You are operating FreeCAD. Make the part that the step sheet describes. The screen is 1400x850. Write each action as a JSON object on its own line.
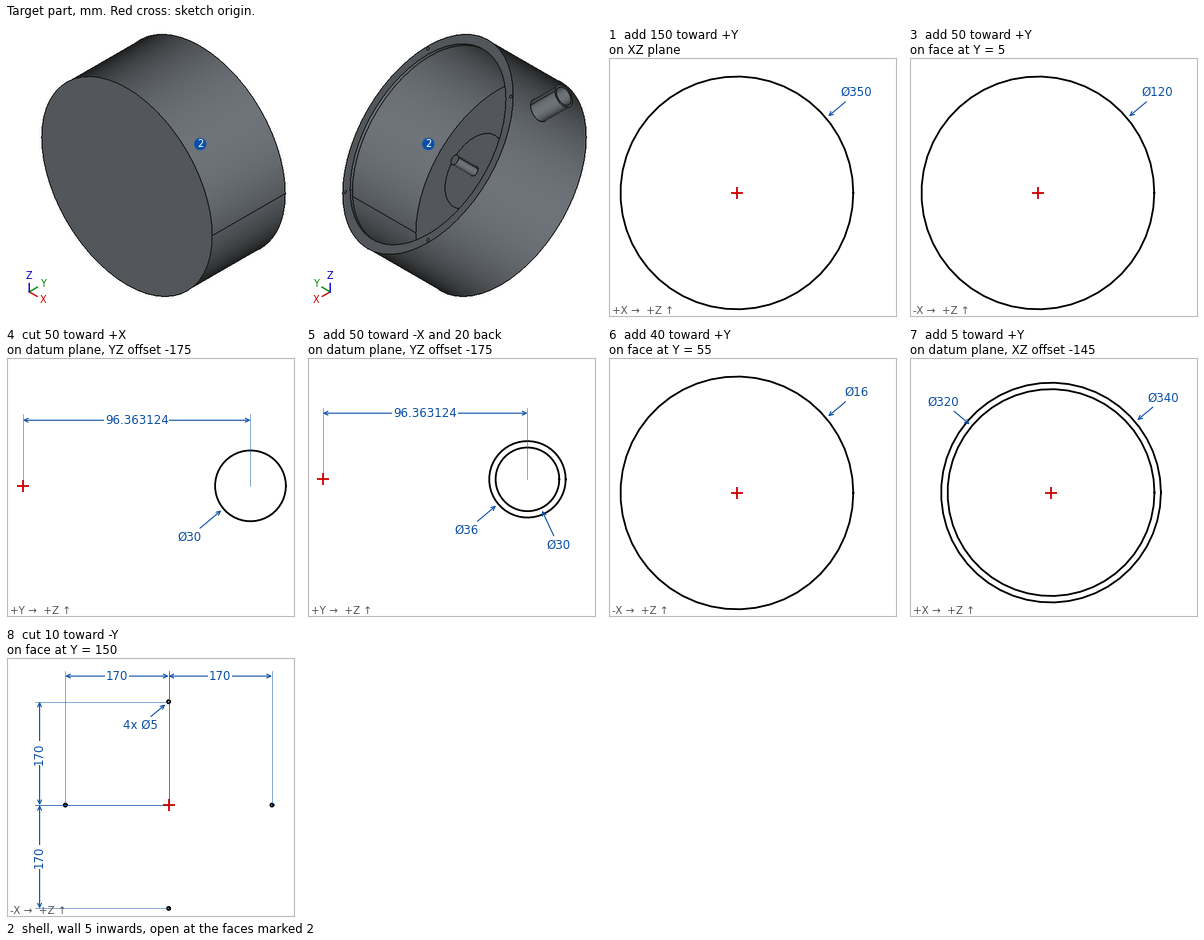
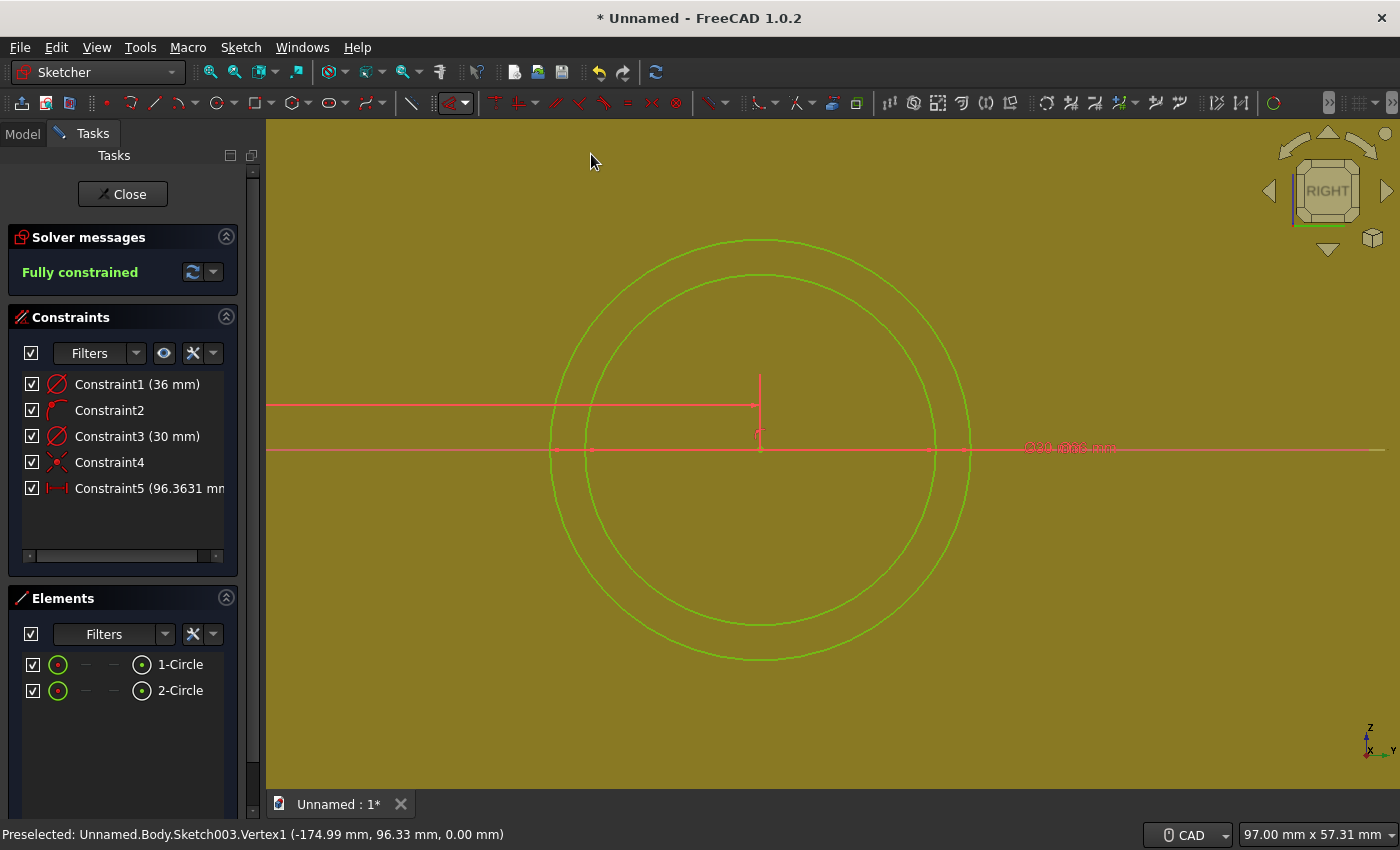
{"action": "left_click", "coordinate": [123, 194]}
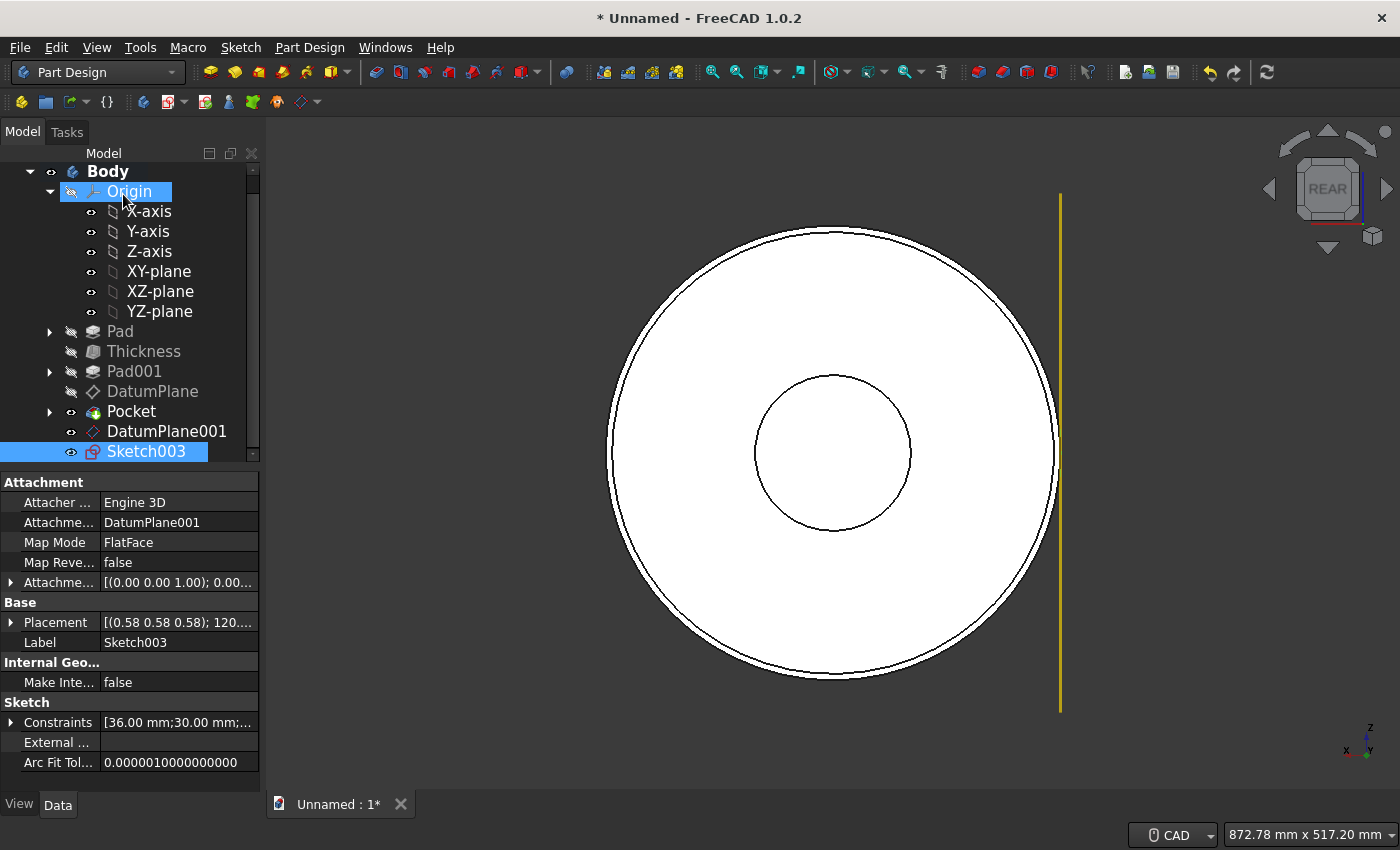
{"action": "left_click", "coordinate": [212, 72]}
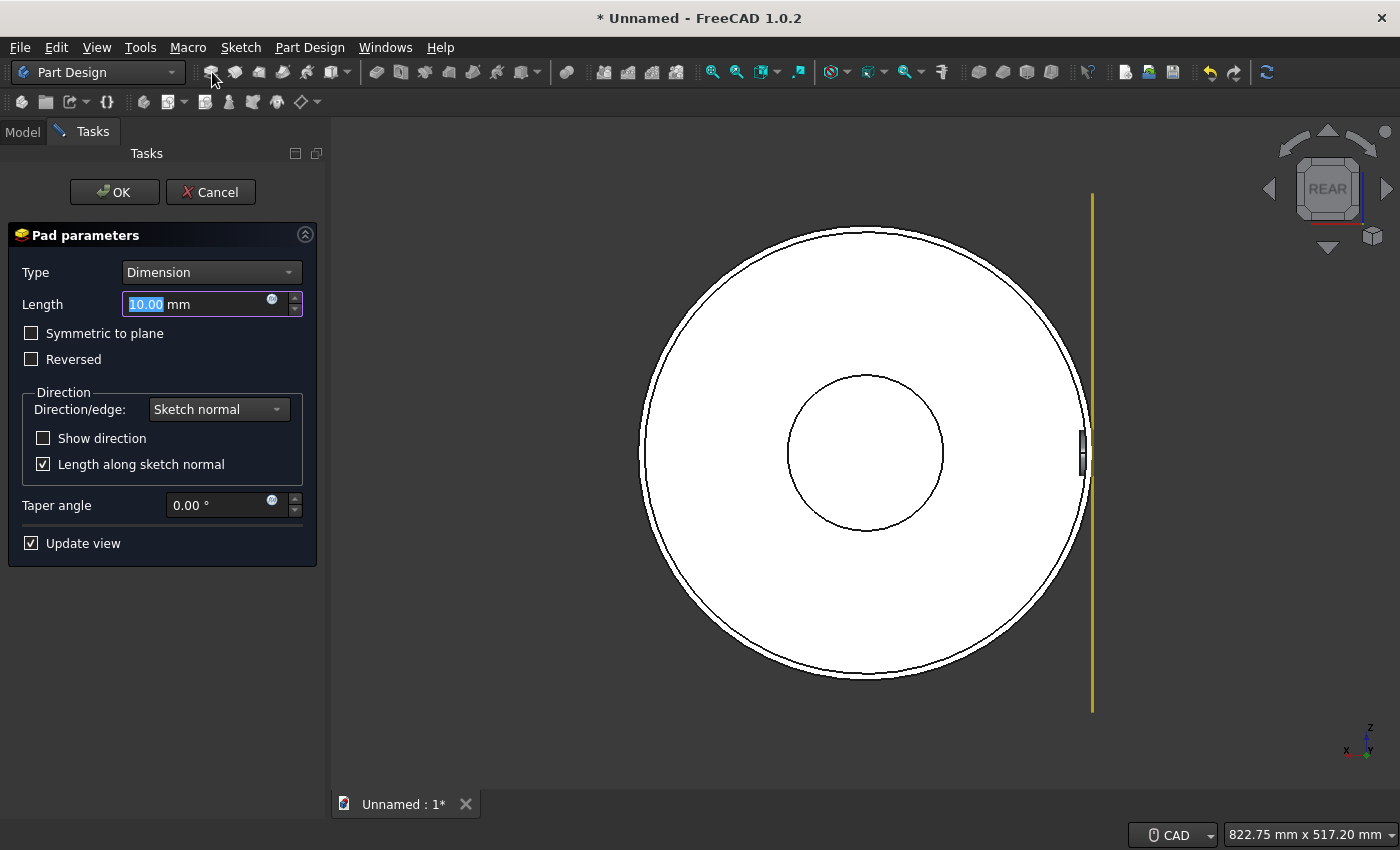
{"action": "left_click", "coordinate": [212, 272]}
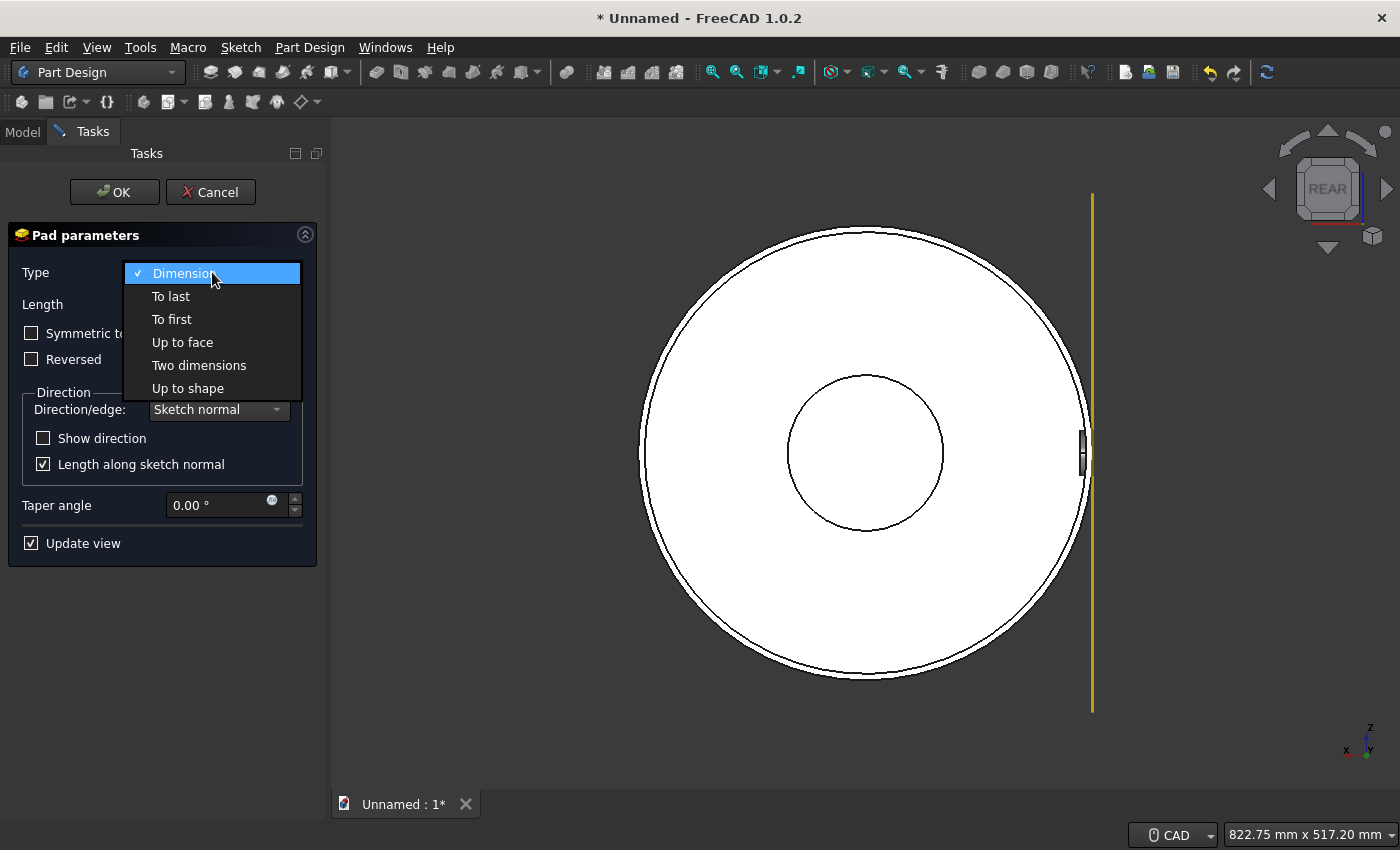
{"action": "left_click", "coordinate": [212, 366]}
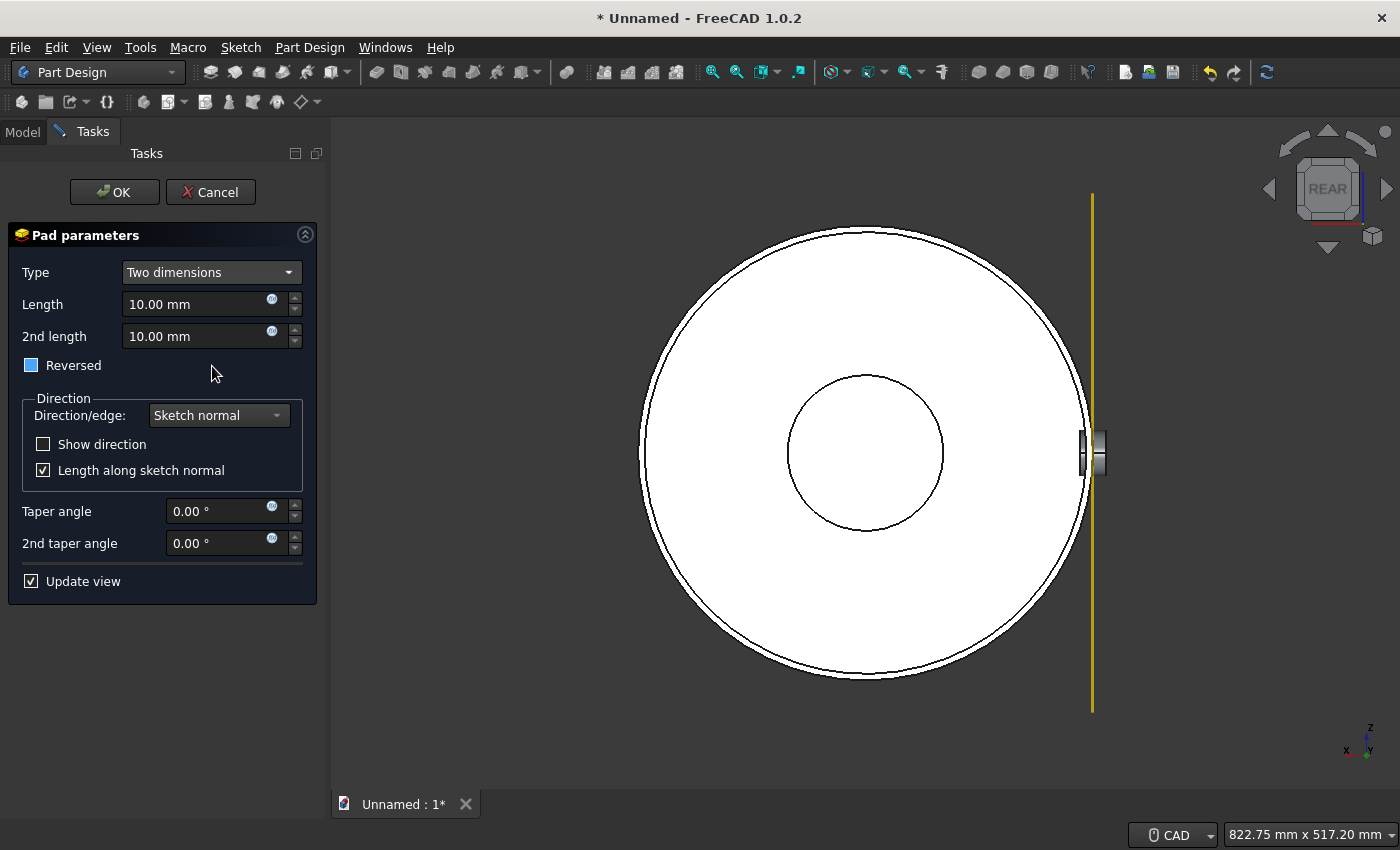
{"action": "triple_click", "coordinate": [204, 304]}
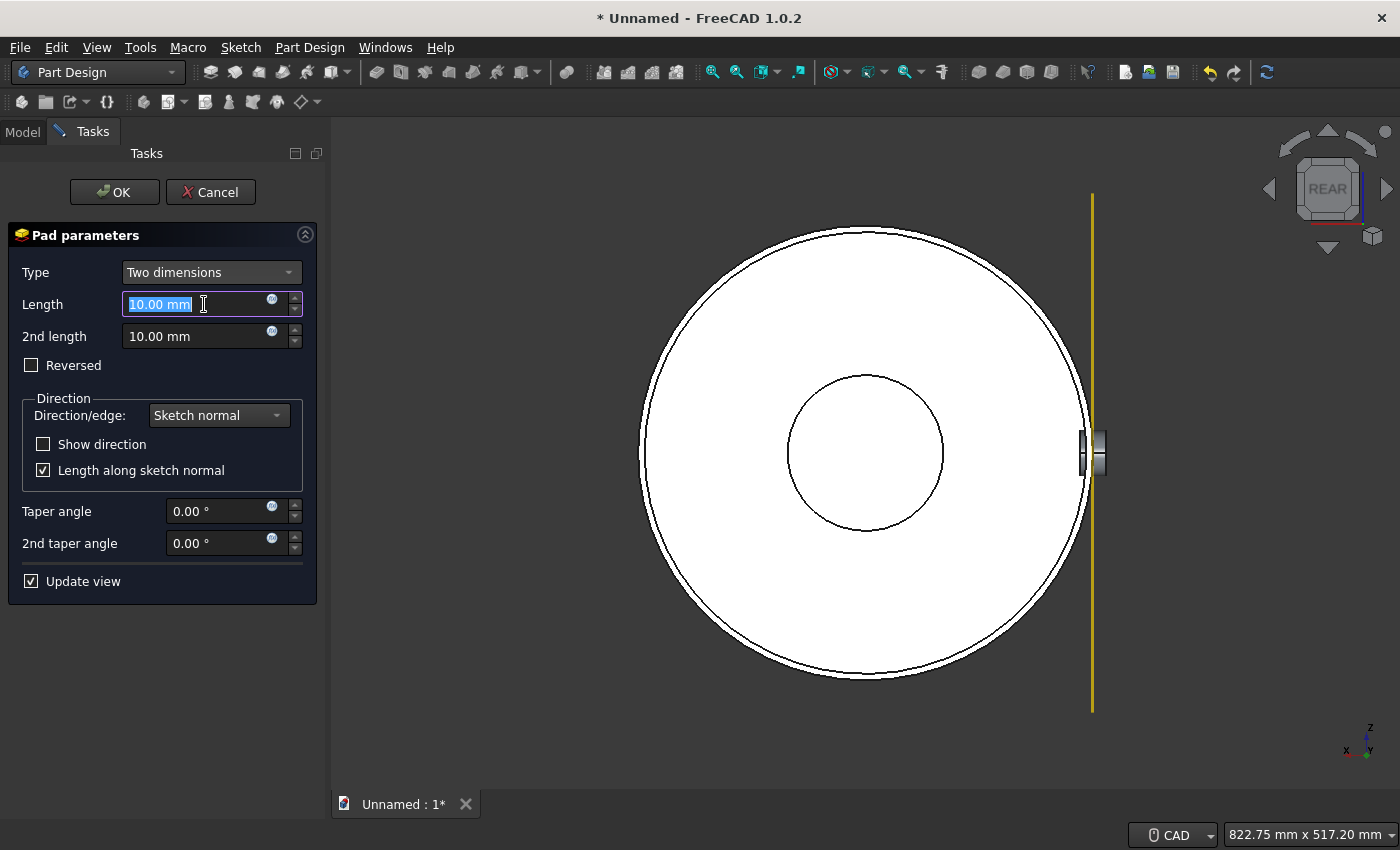
{"action": "type", "text": "50"}
{"action": "key", "text": "Tab"}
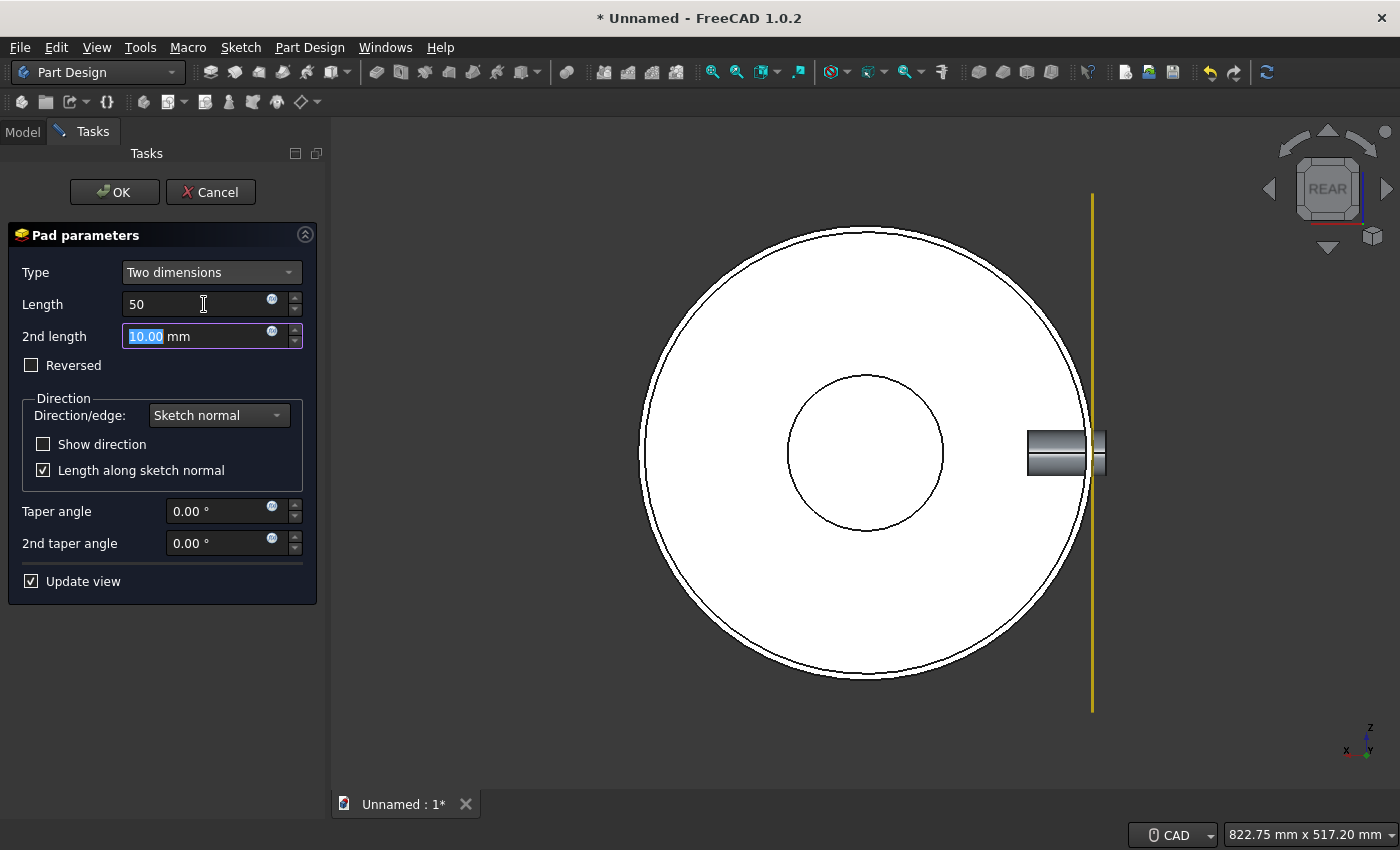
{"action": "type", "text": "20"}
{"action": "key", "text": "Tab"}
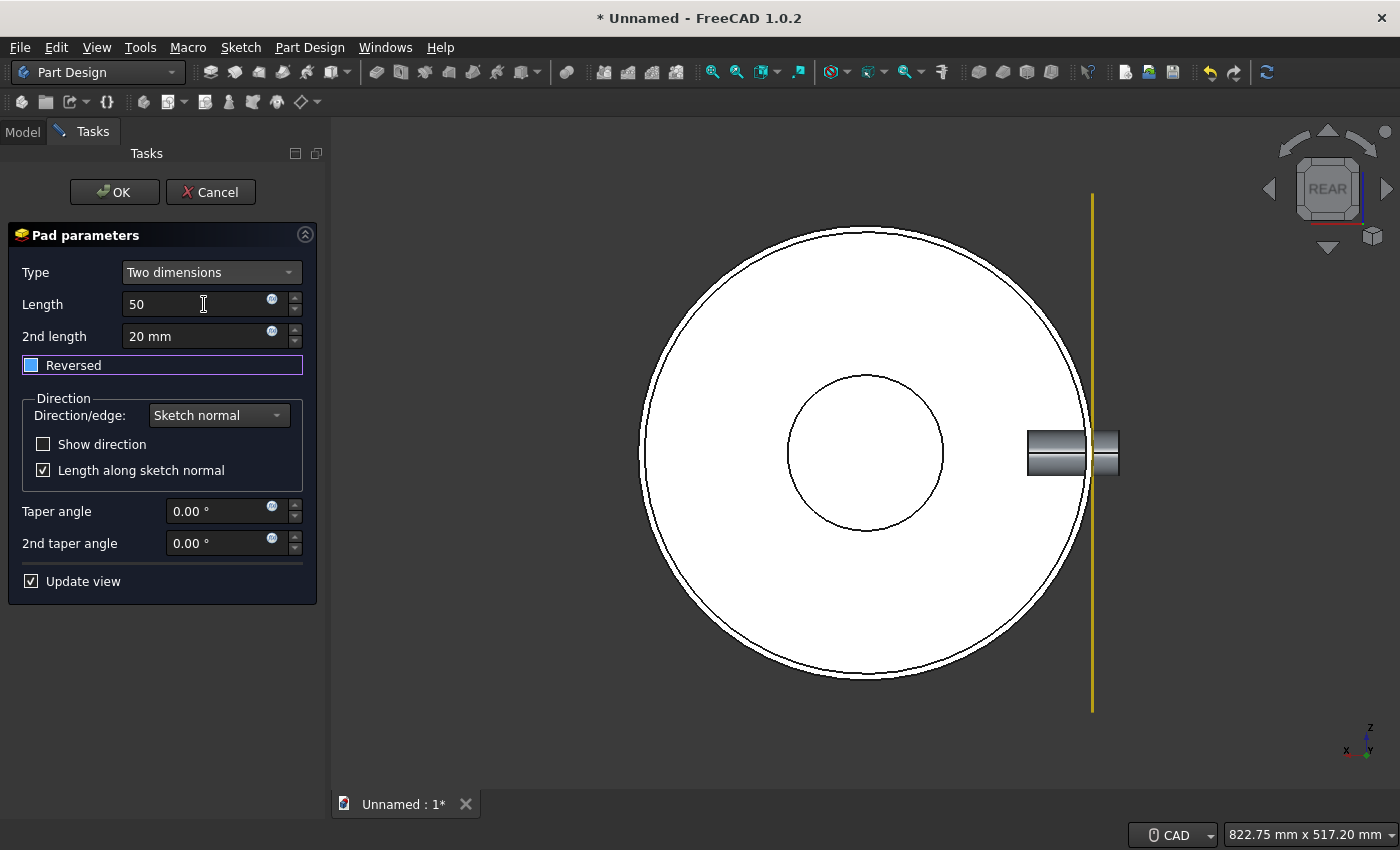
{"action": "left_click", "coordinate": [30, 365]}